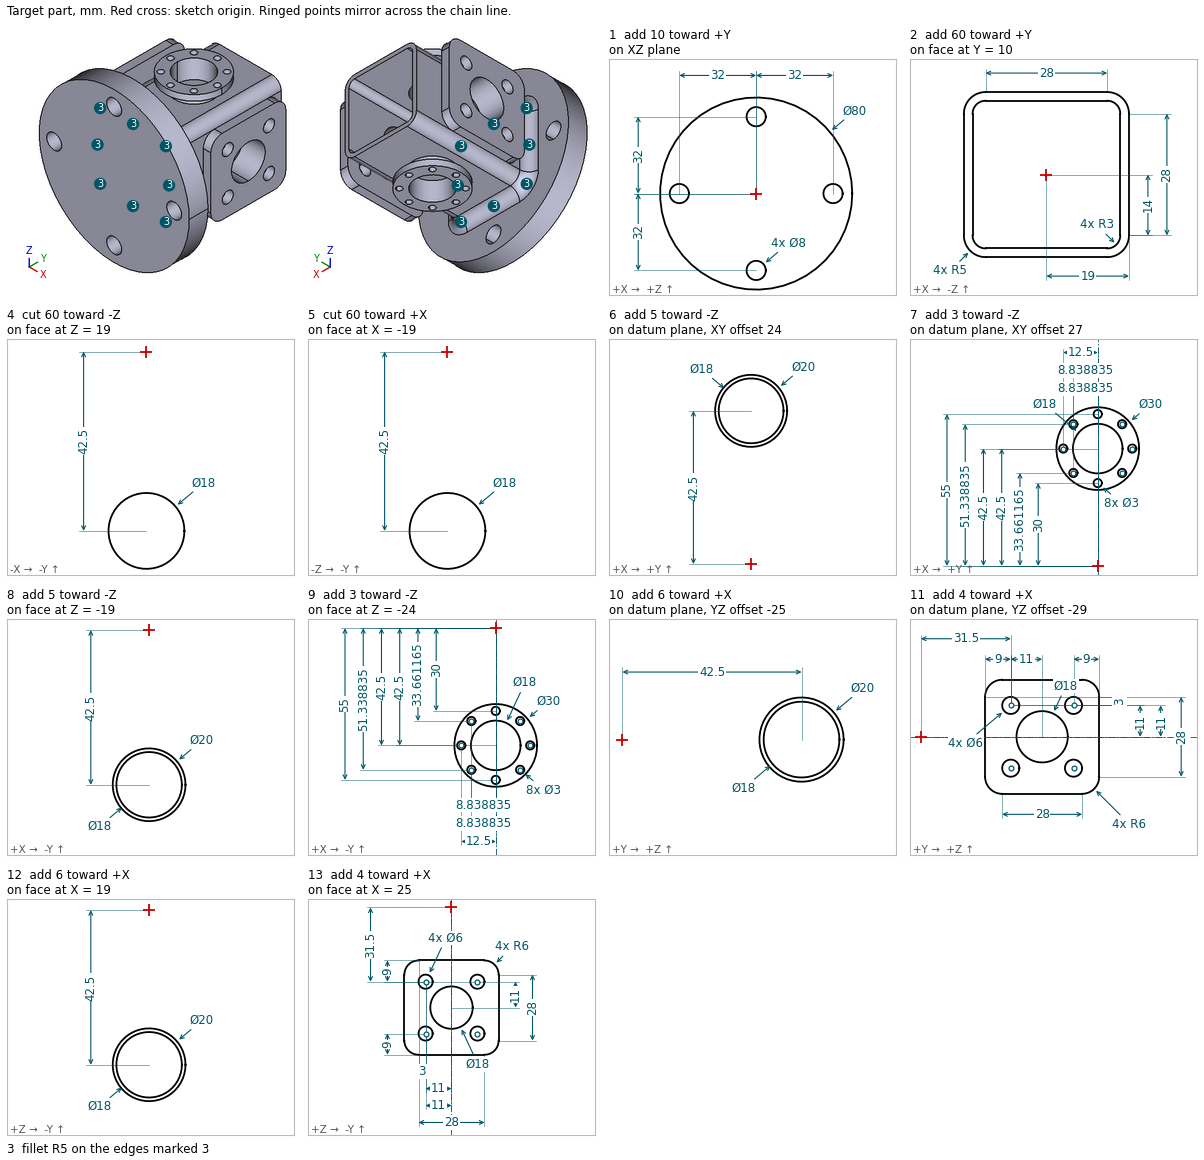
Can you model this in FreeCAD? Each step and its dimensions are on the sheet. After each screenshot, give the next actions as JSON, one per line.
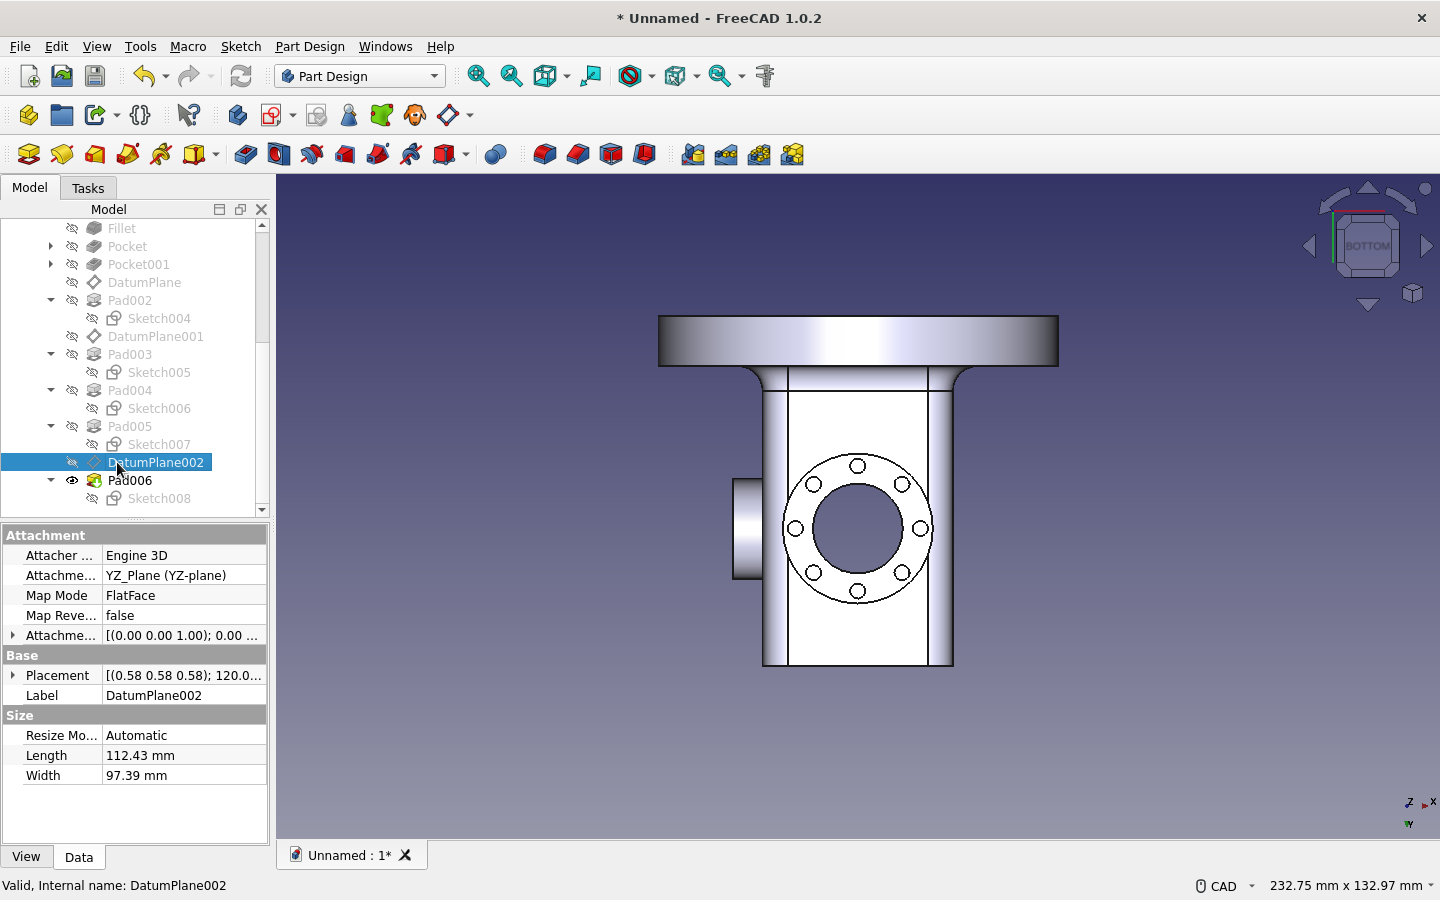
{"action": "scroll", "coordinate": [141, 368], "scroll_direction": "down", "scroll_amount": 3}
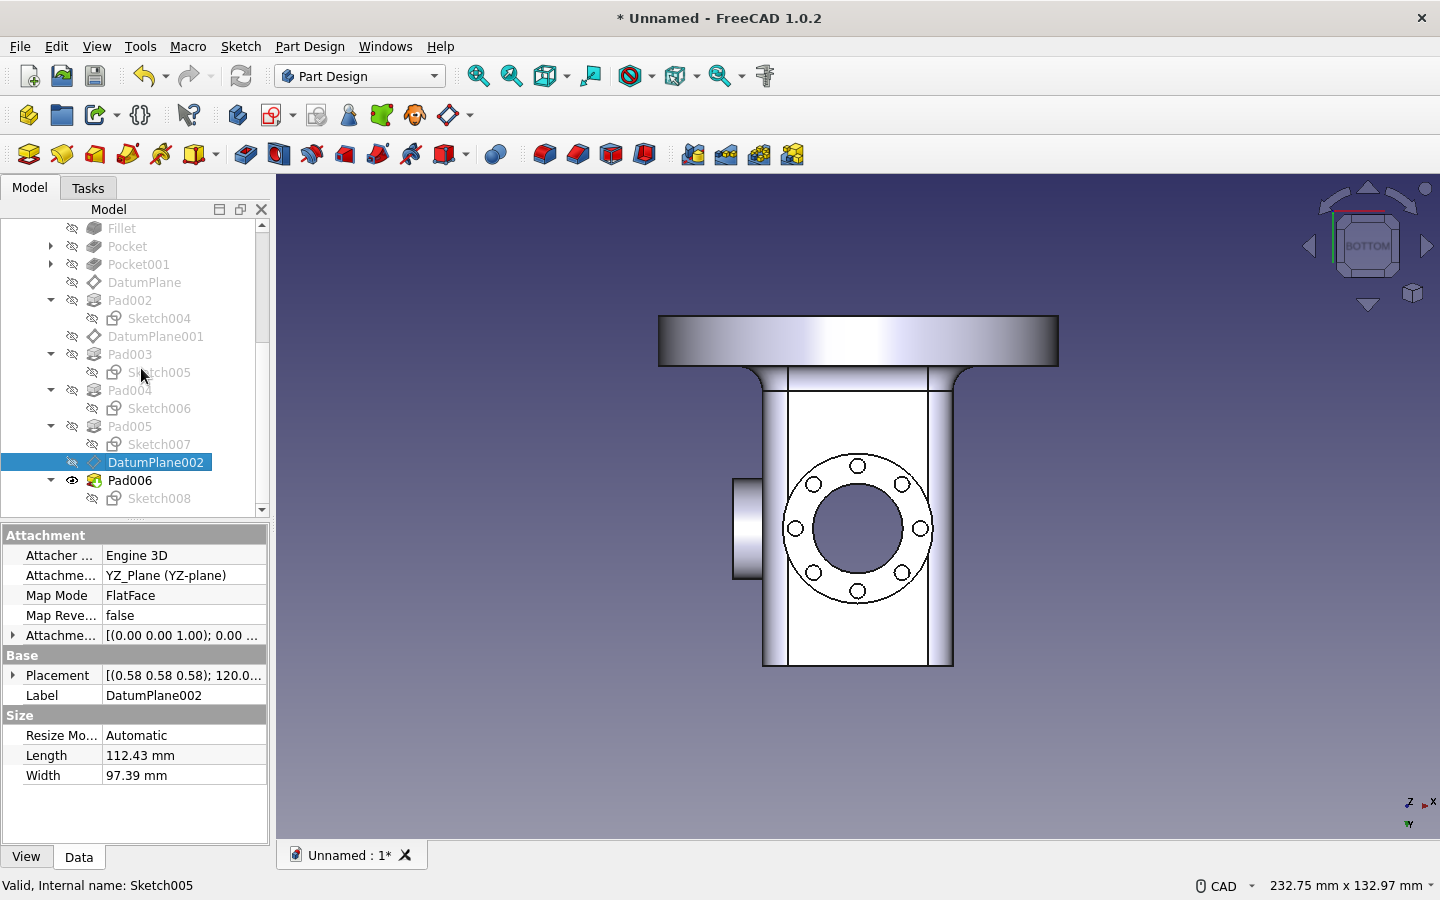
{"action": "scroll", "coordinate": [141, 368], "scroll_direction": "up", "scroll_amount": 15}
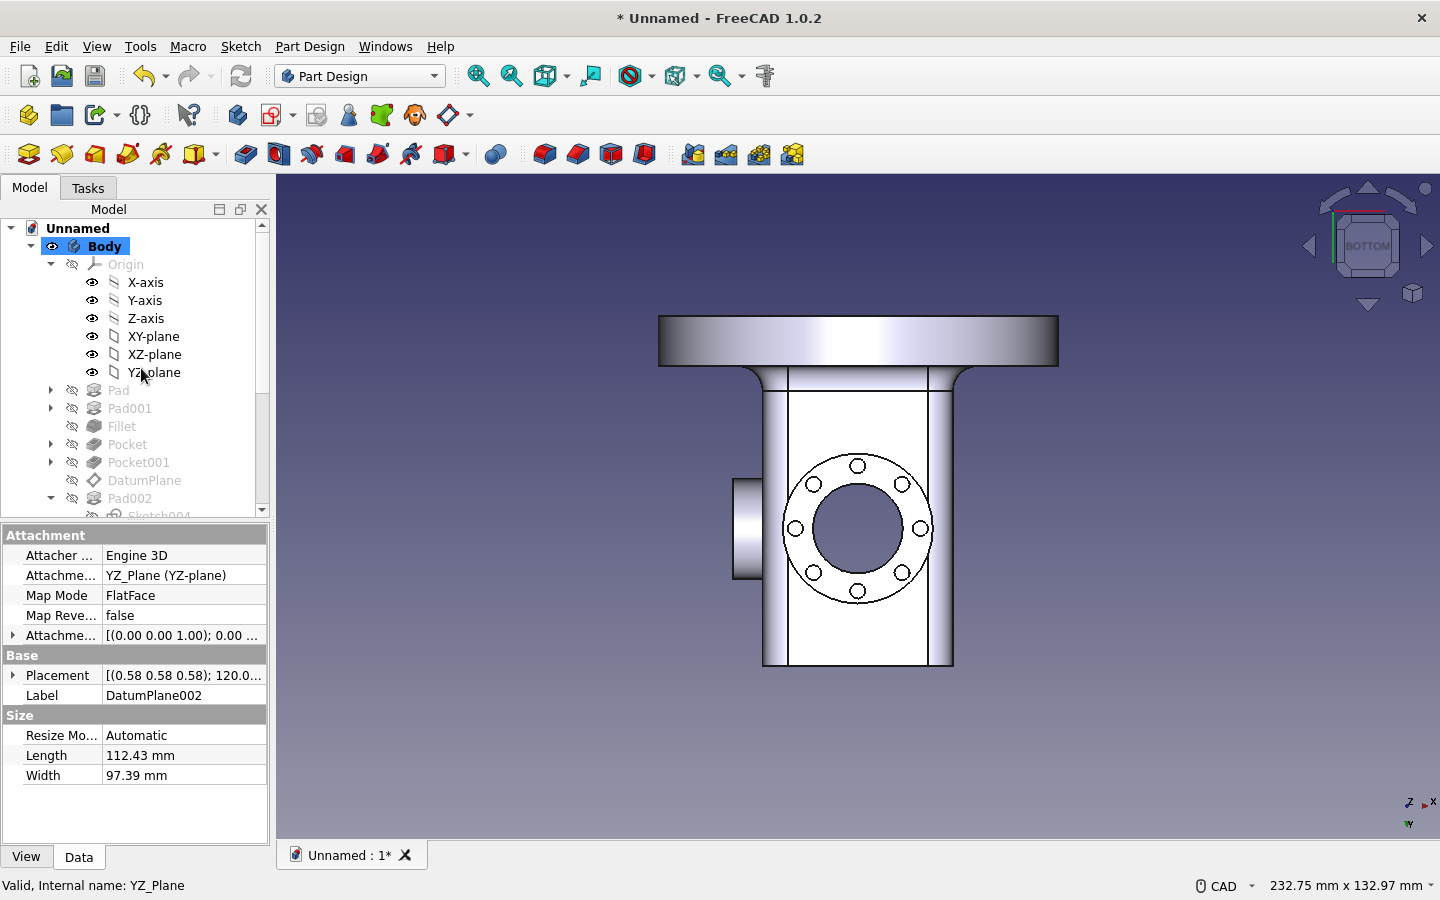
{"action": "left_click", "coordinate": [137, 372]}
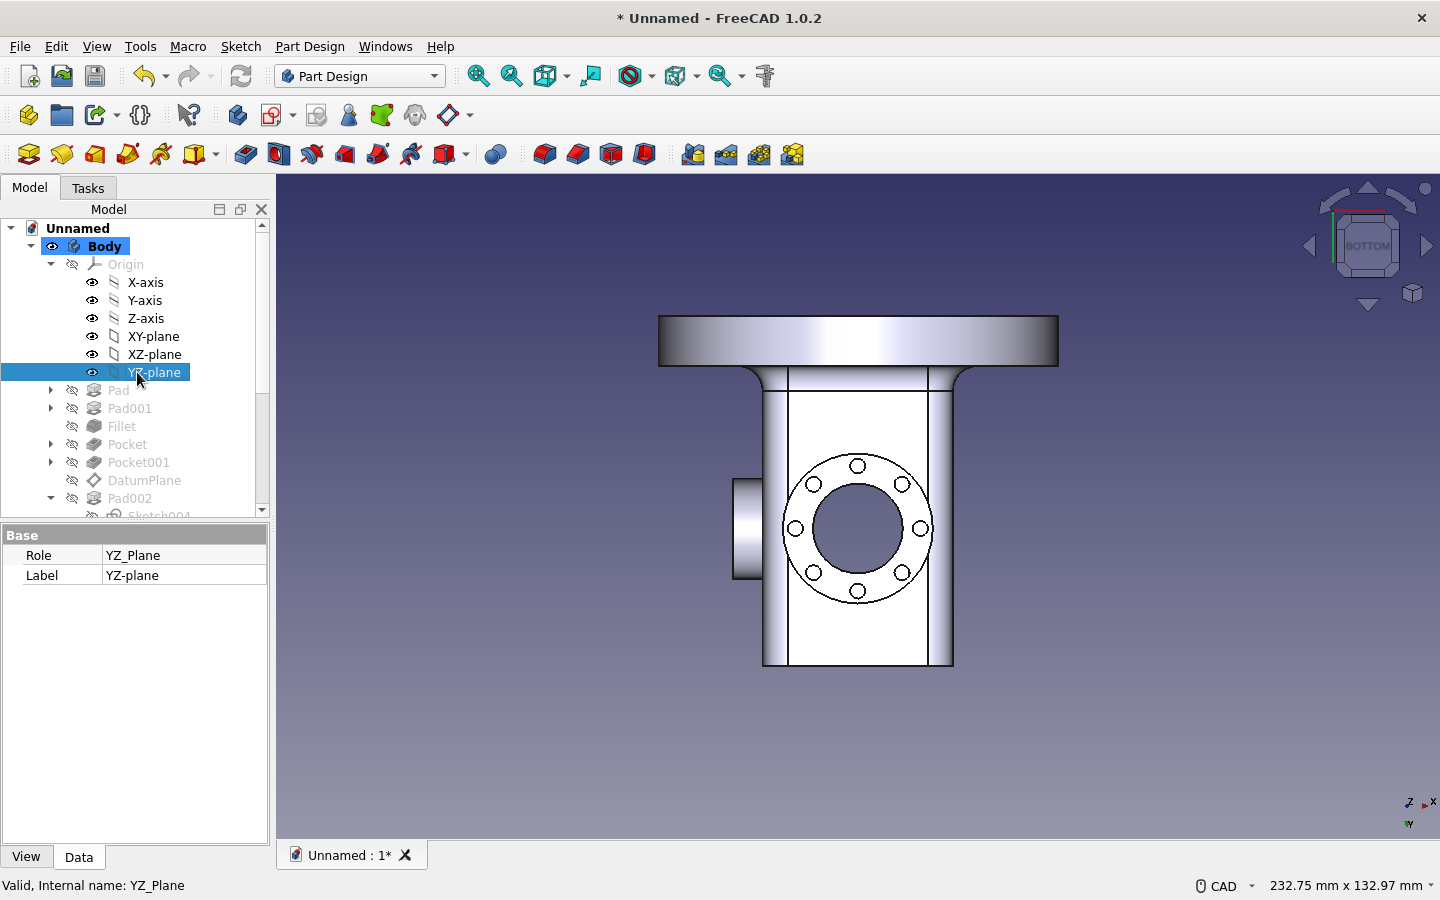
{"action": "left_click", "coordinate": [448, 116]}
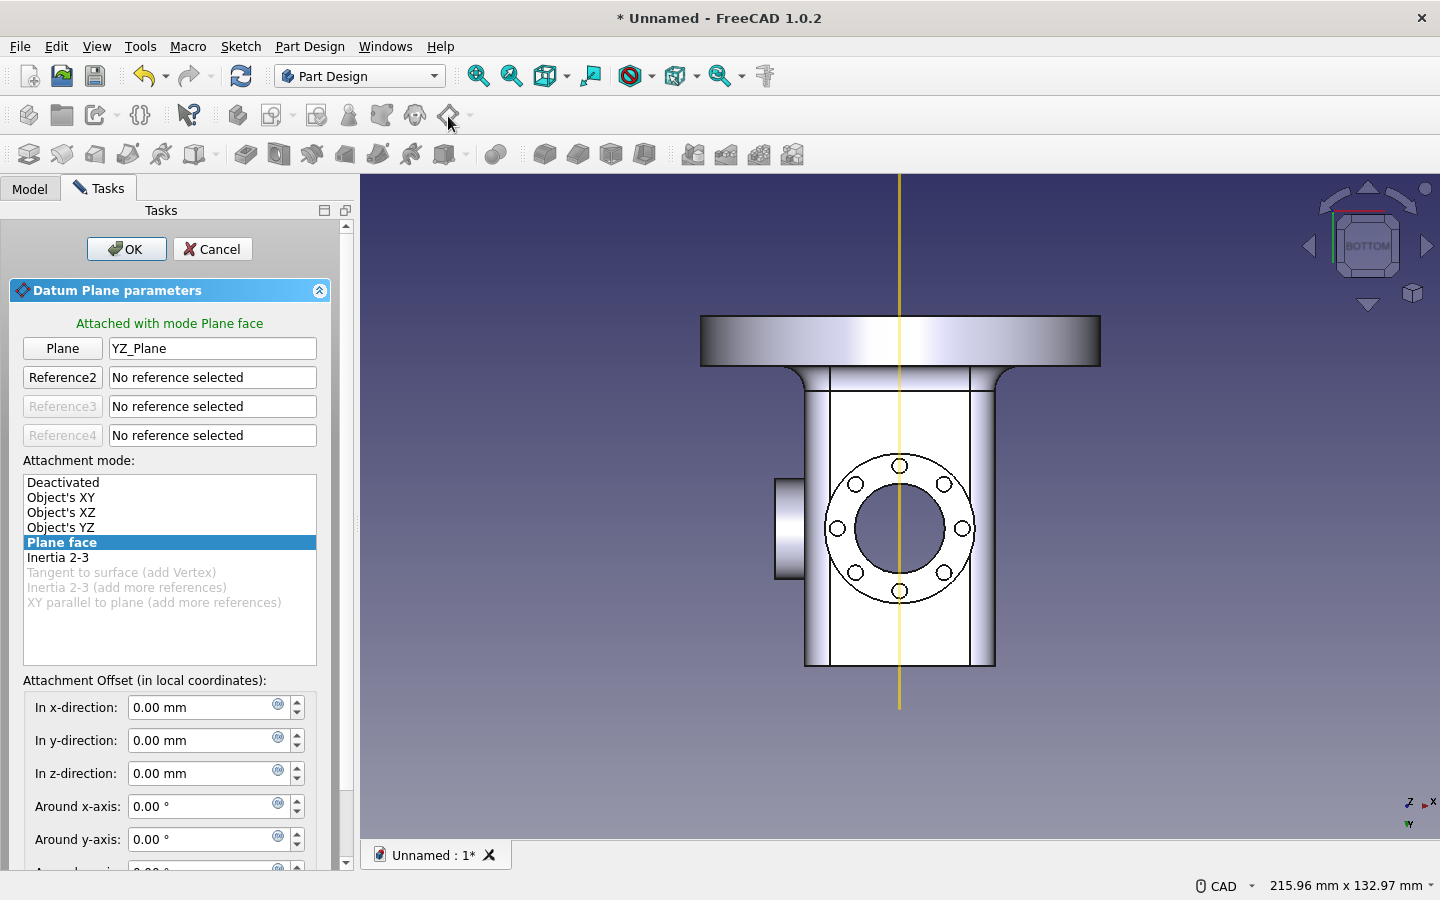
{"action": "triple_click", "coordinate": [210, 774]}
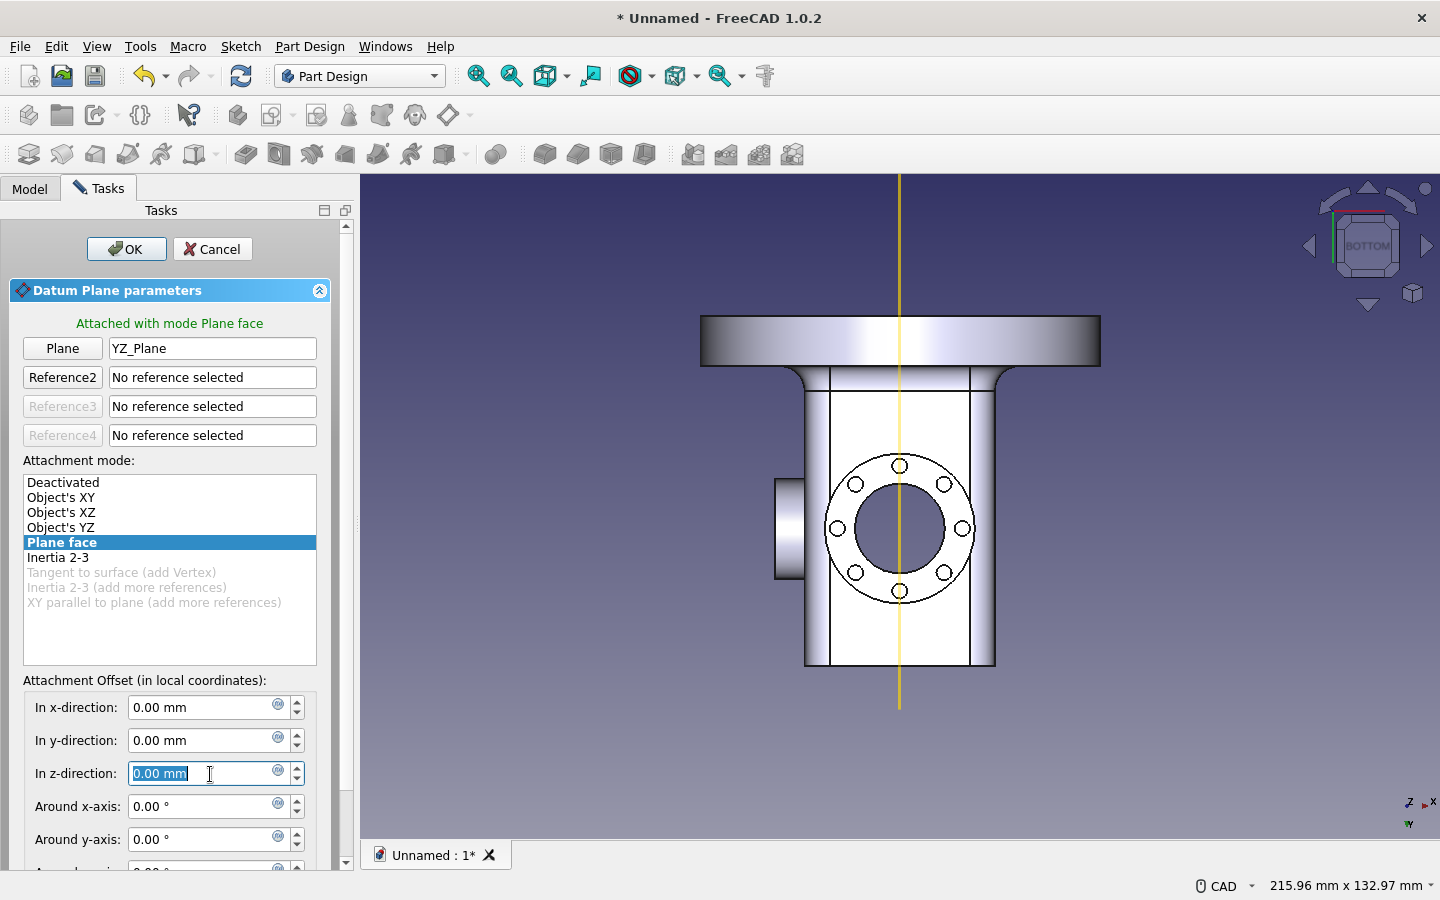
{"action": "type", "text": "-29"}
{"action": "key", "text": "Tab"}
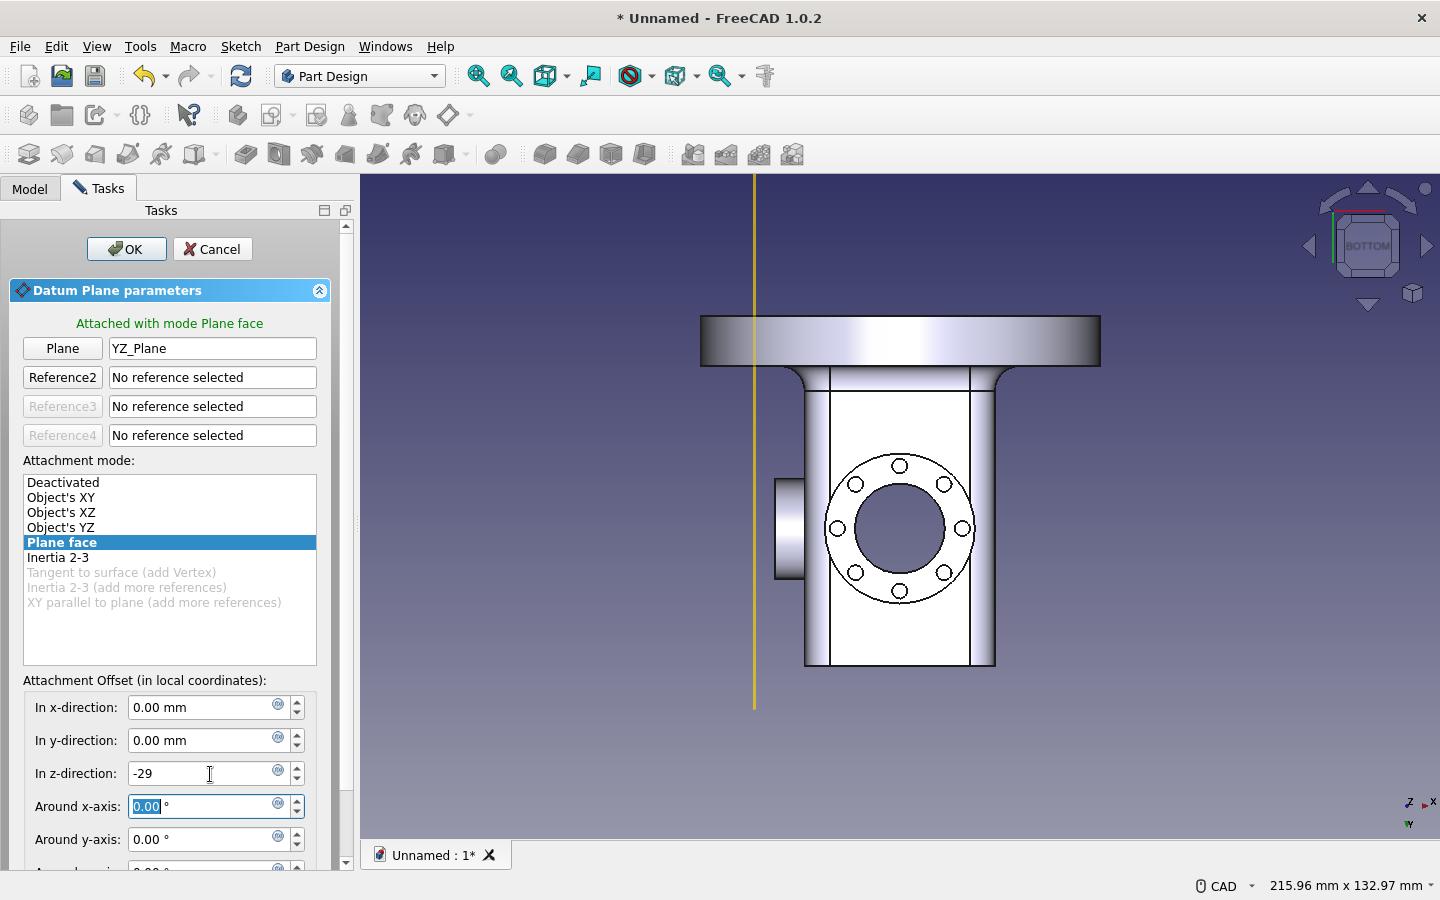
{"action": "left_click", "coordinate": [127, 249]}